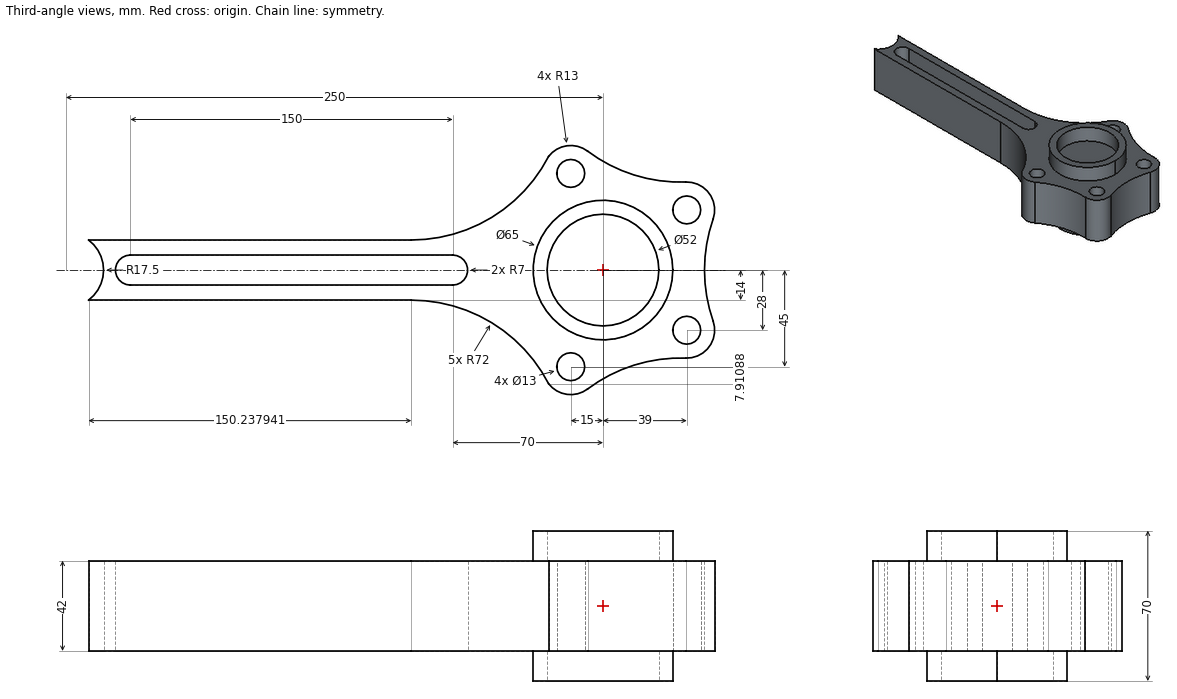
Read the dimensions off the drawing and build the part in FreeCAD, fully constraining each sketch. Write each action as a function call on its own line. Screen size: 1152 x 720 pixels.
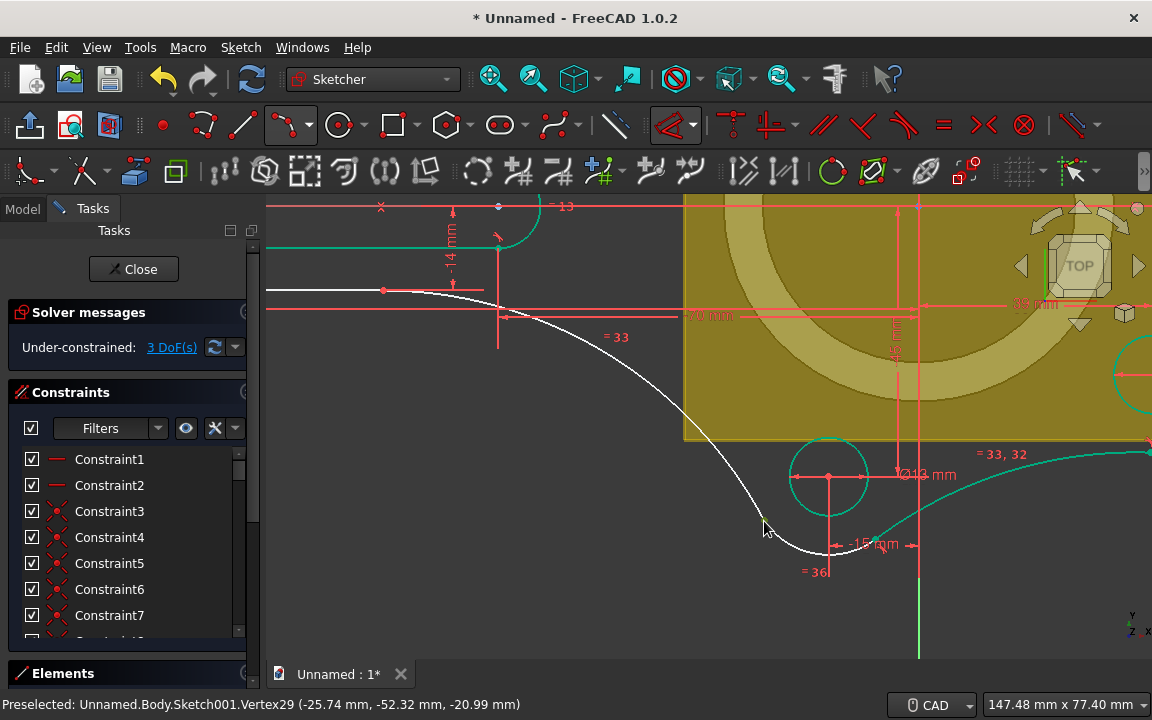
click(829, 477)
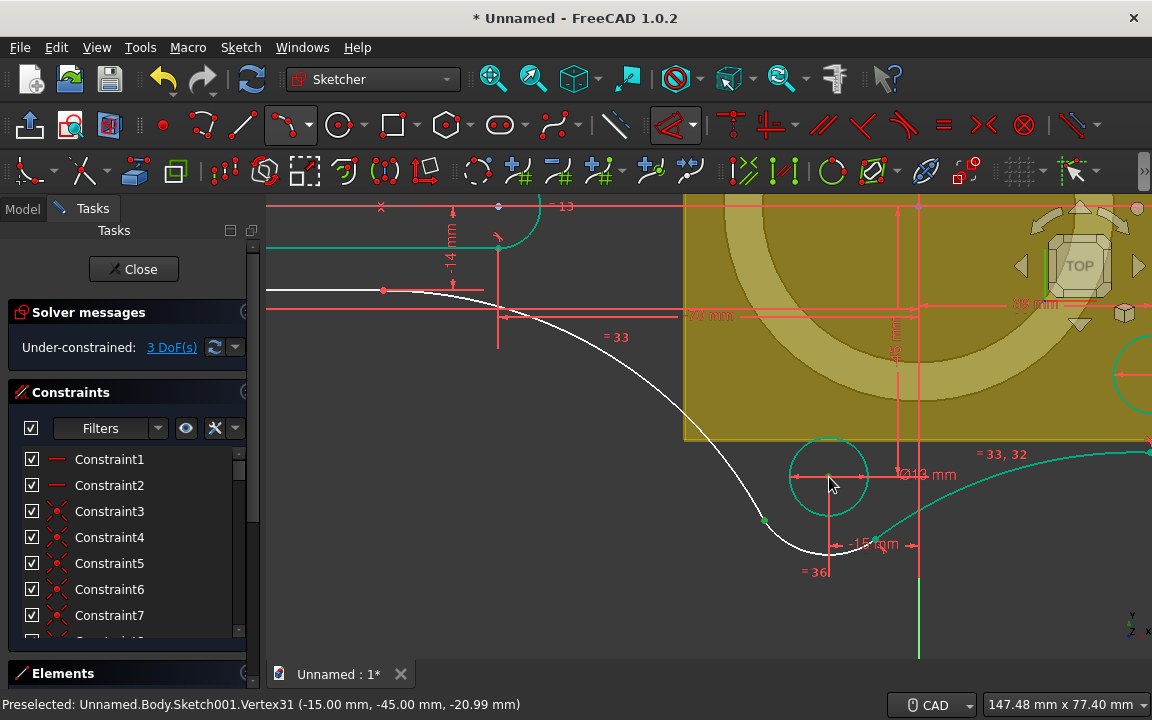
key(i)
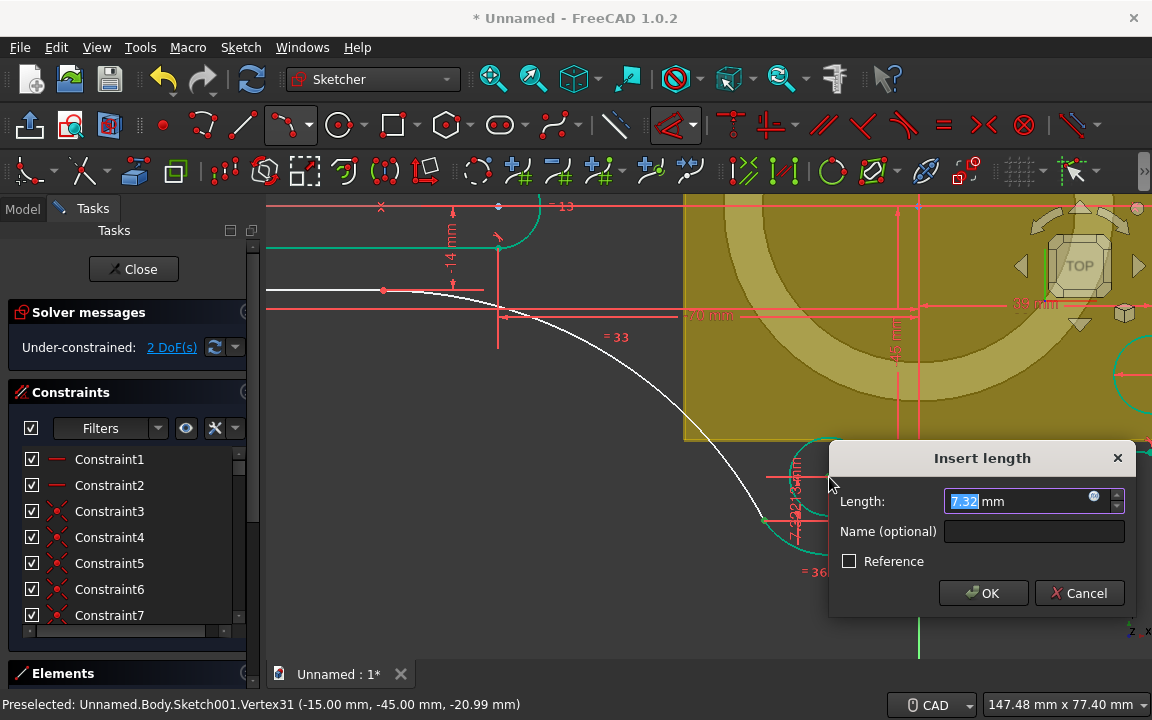
text(7.91088)
key(Return)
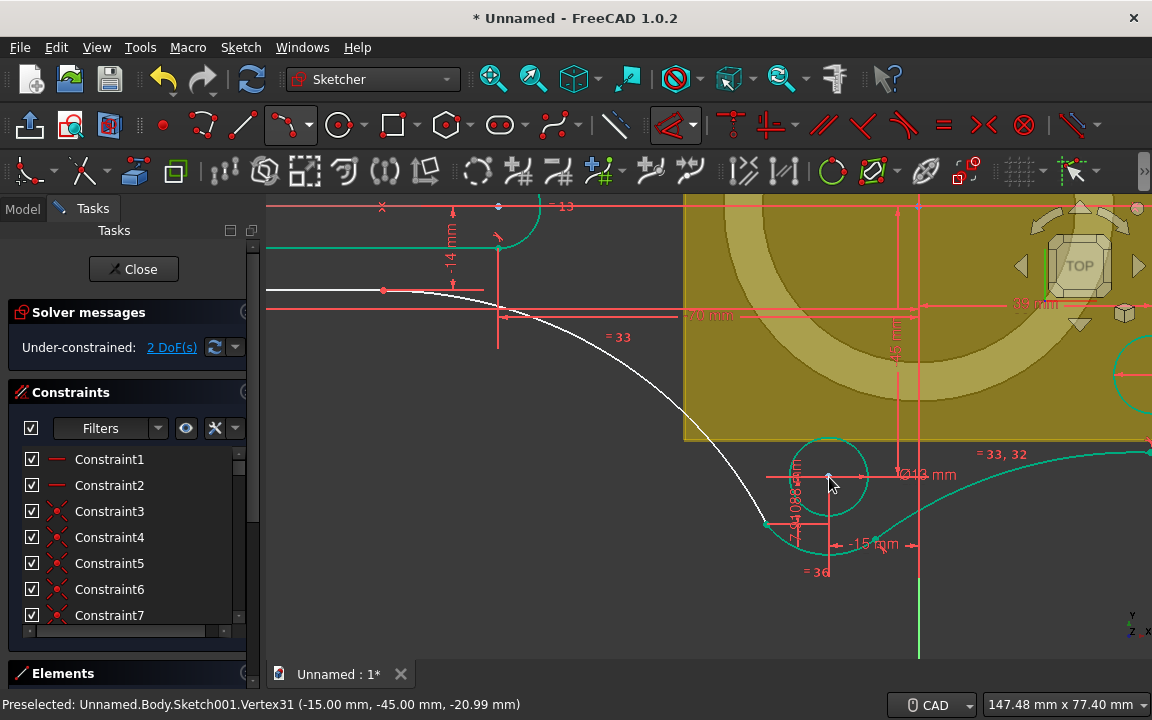
scroll(764, 521, down, 6)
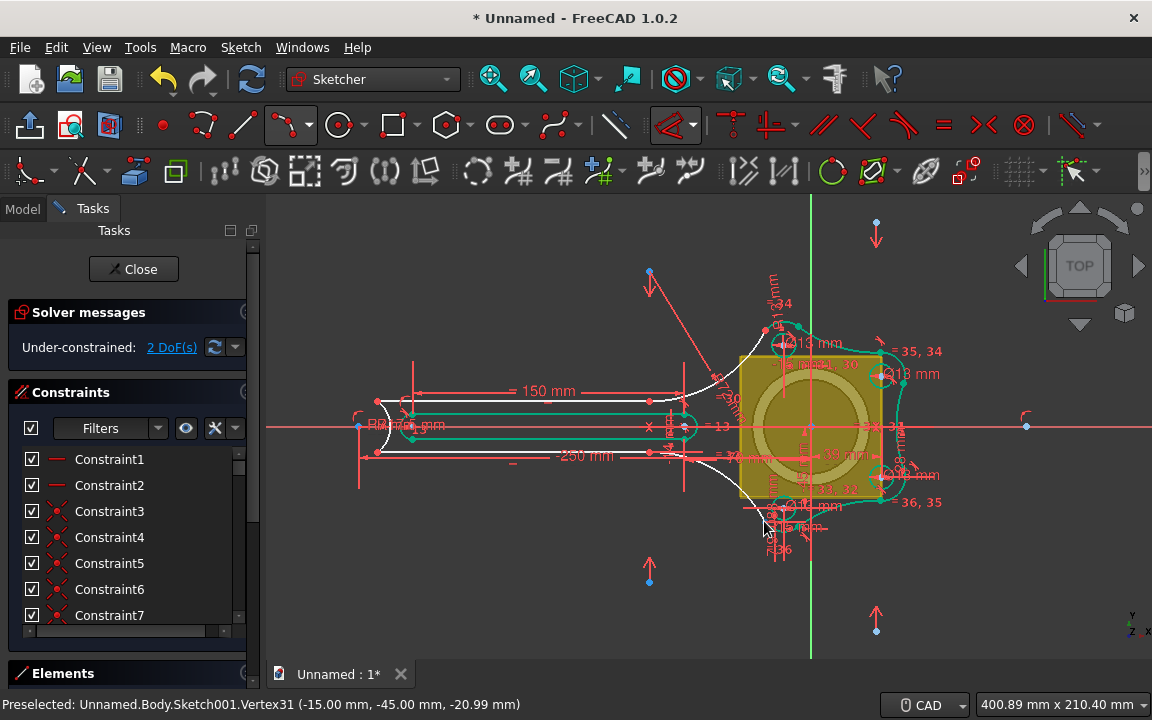
click(459, 452)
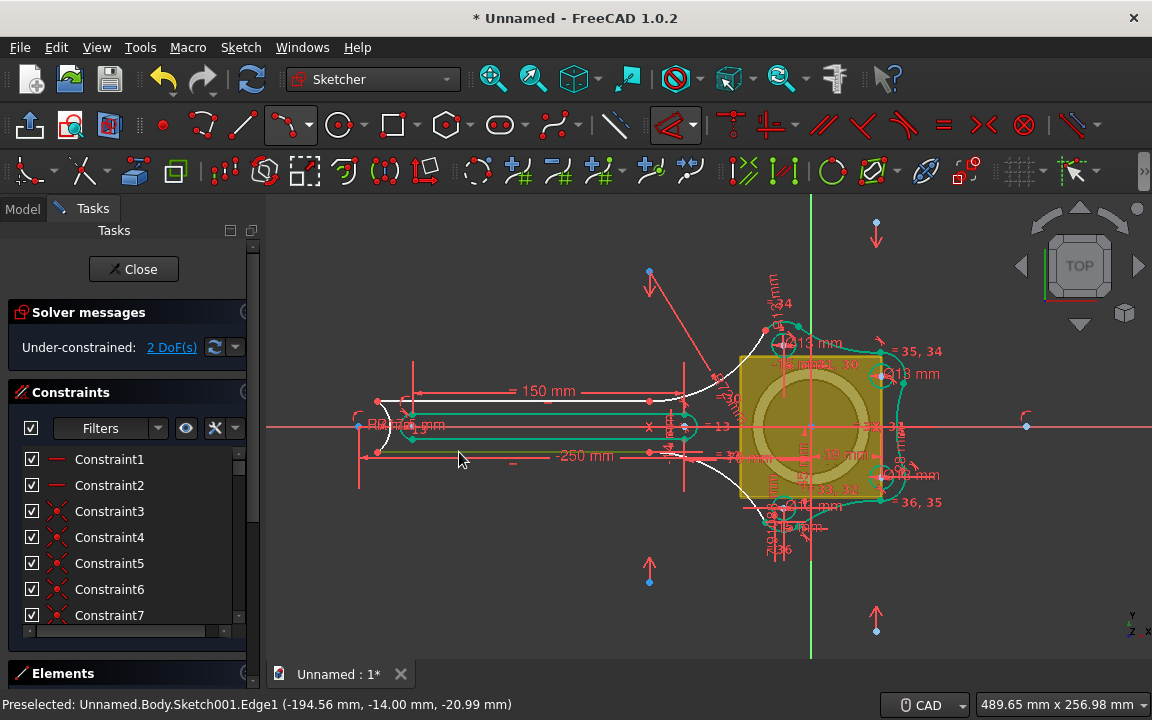
key(l)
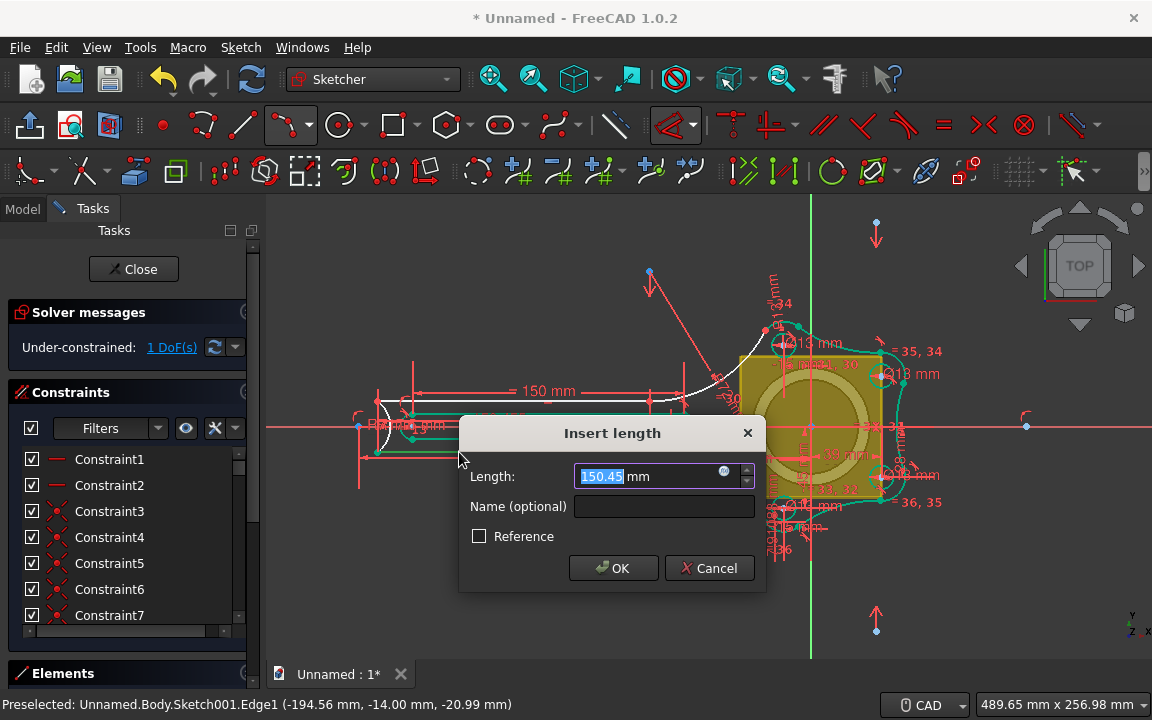
text(150.237941)
key(Return)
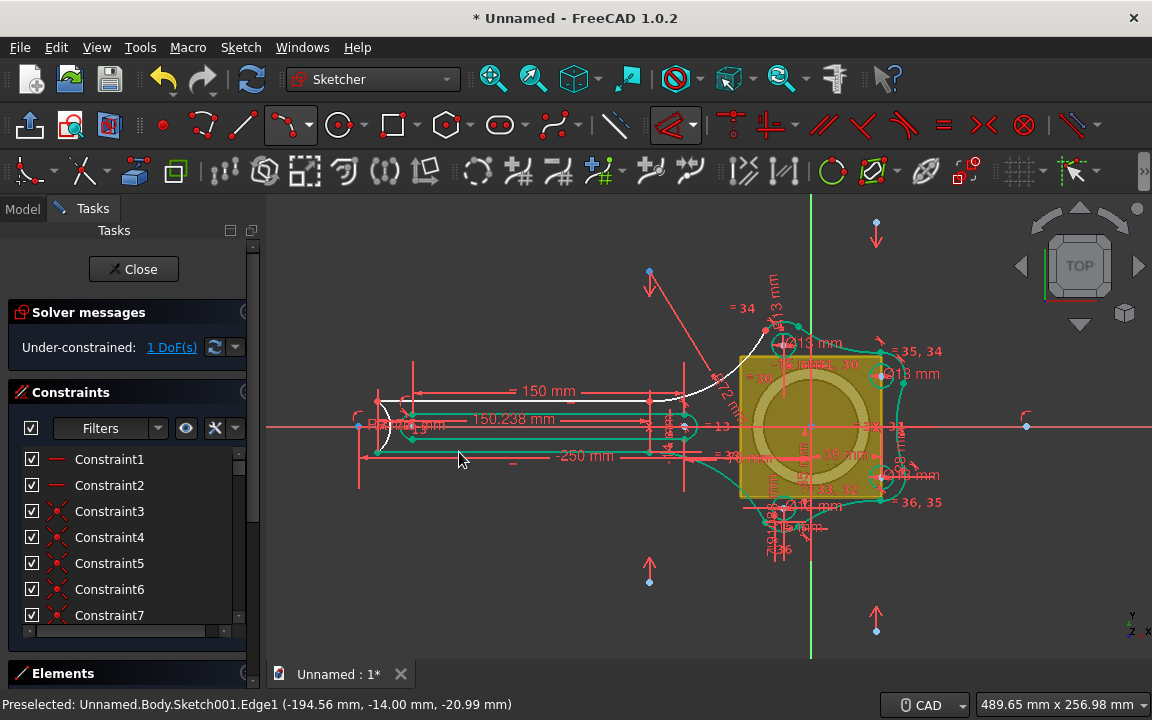
click(459, 401)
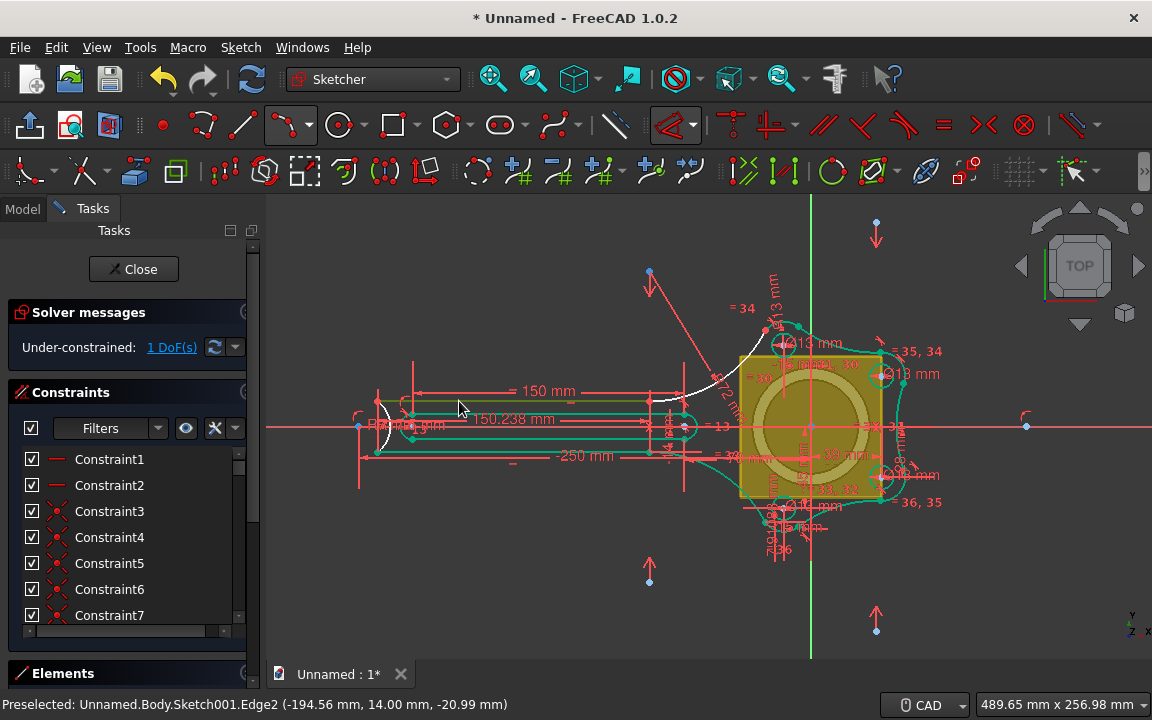
click(696, 126)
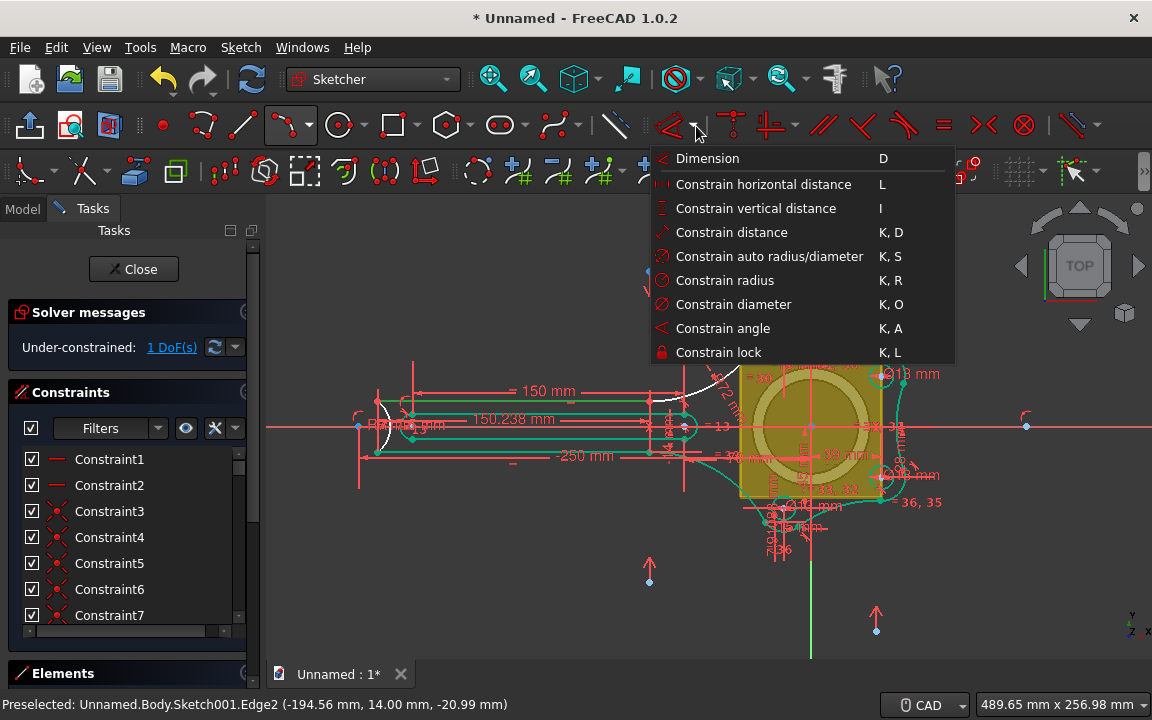
click(803, 184)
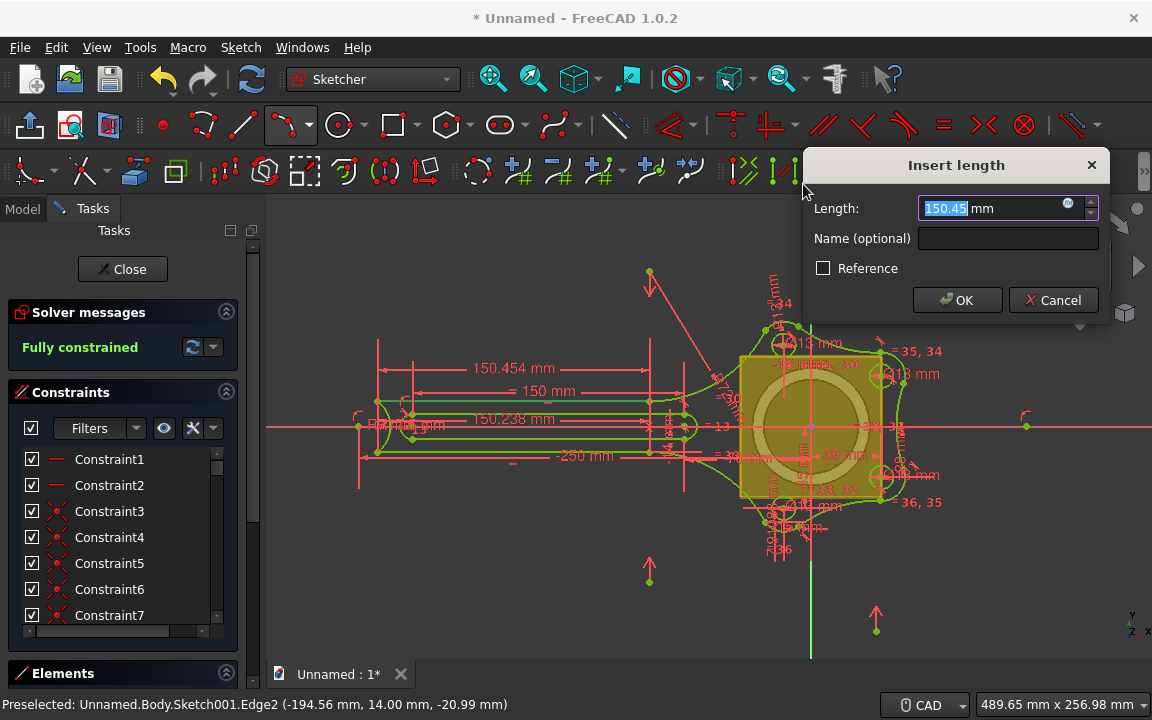
text(150.237941)
key(Return)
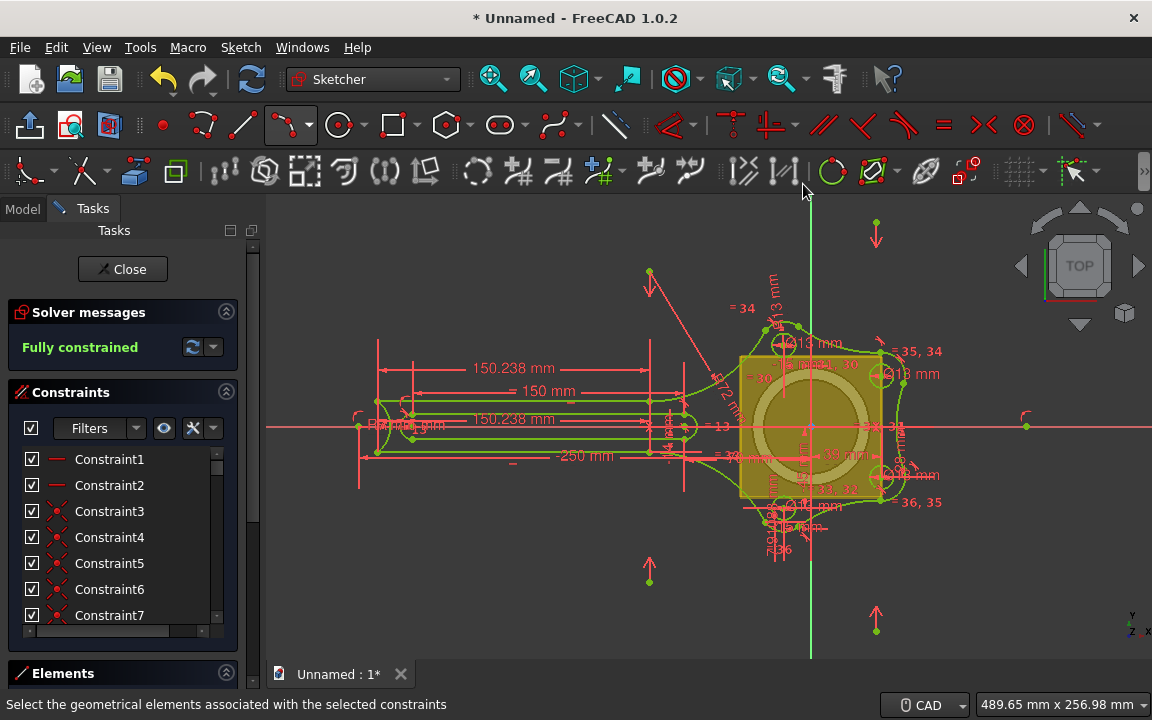
click(123, 269)